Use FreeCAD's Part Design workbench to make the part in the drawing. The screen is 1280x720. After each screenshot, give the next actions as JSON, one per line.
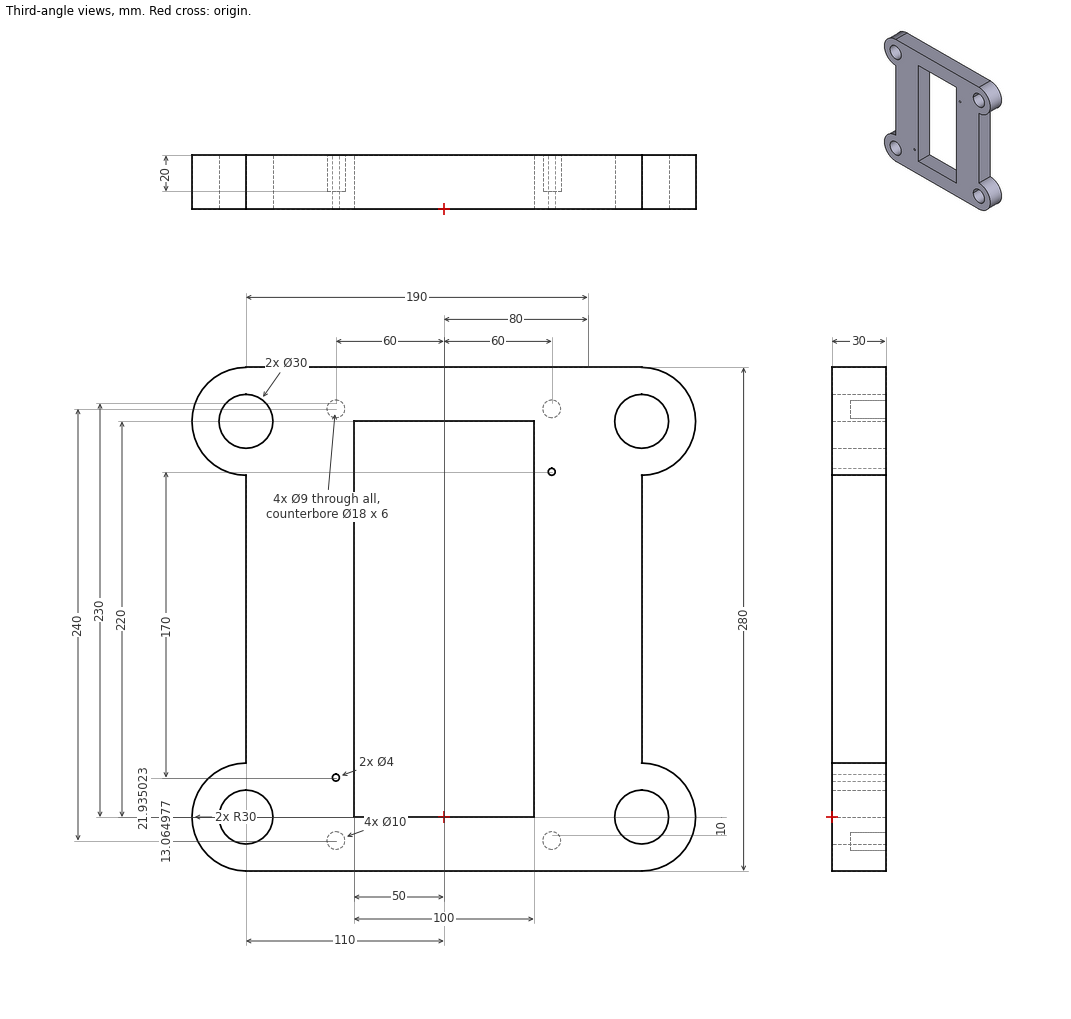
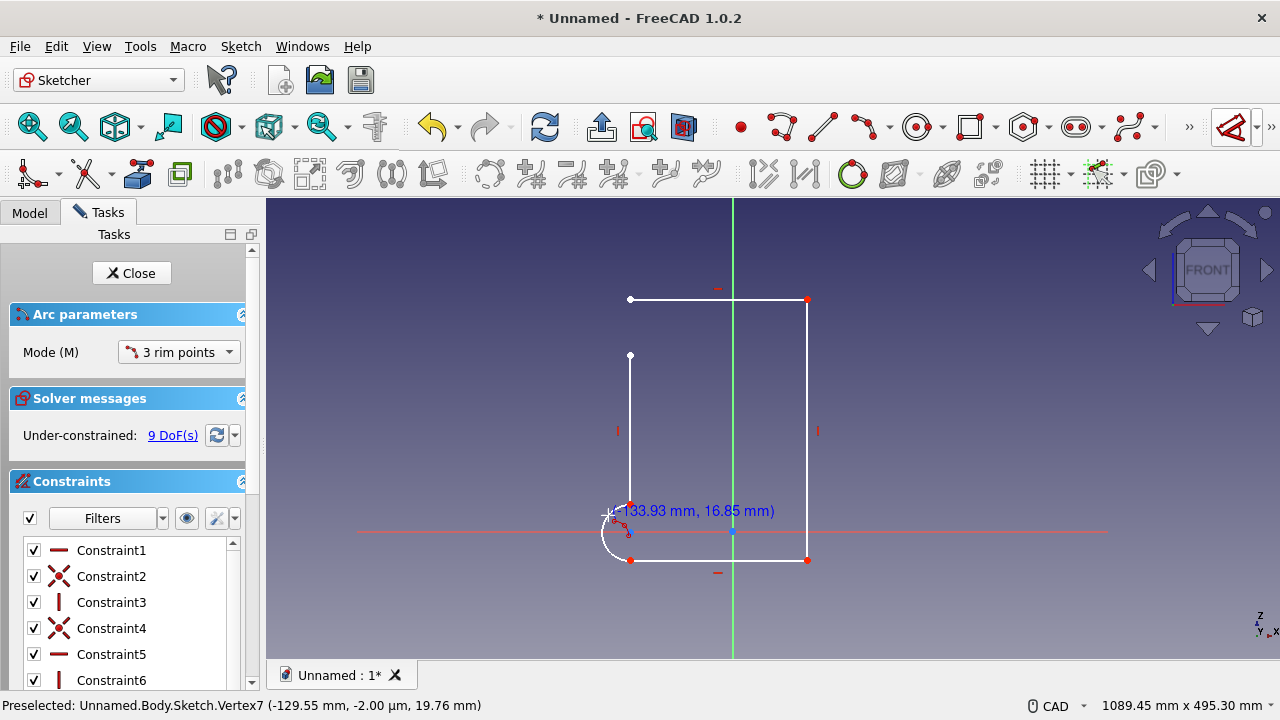
{"action": "left_click", "coordinate": [630, 356]}
{"action": "left_click", "coordinate": [630, 300]}
{"action": "left_click", "coordinate": [602, 327]}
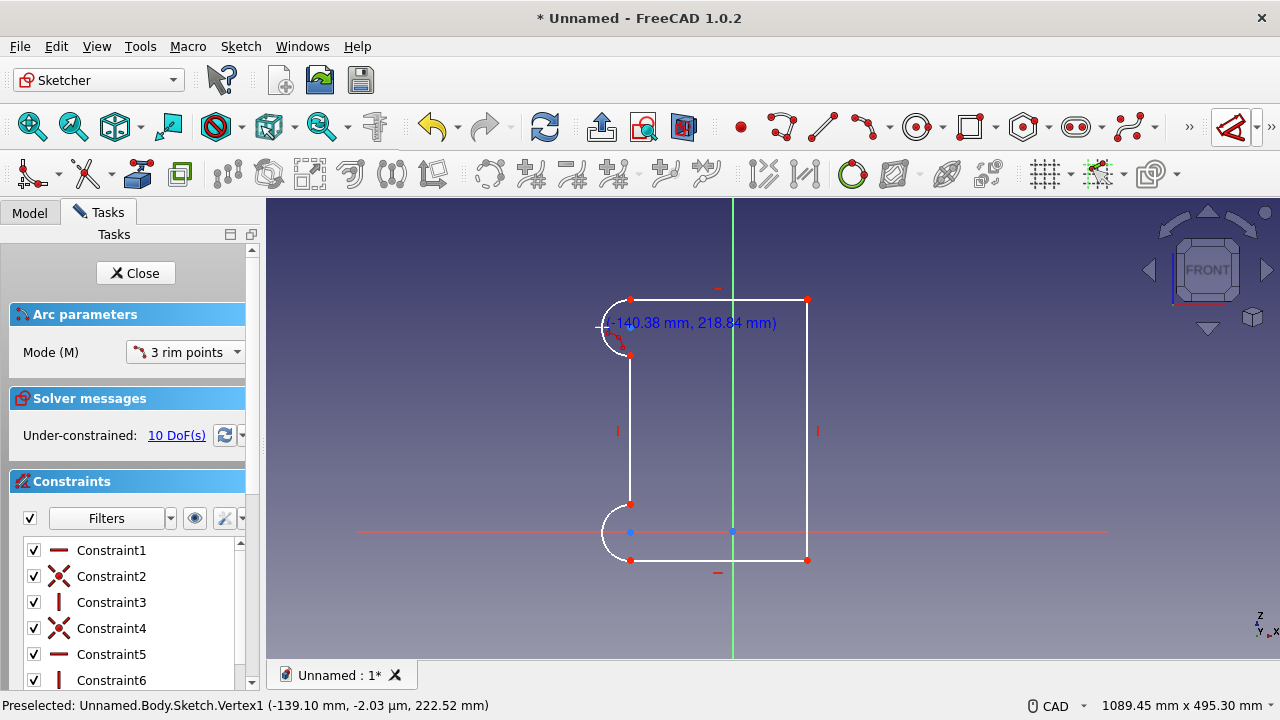
{"action": "left_click", "coordinate": [970, 128]}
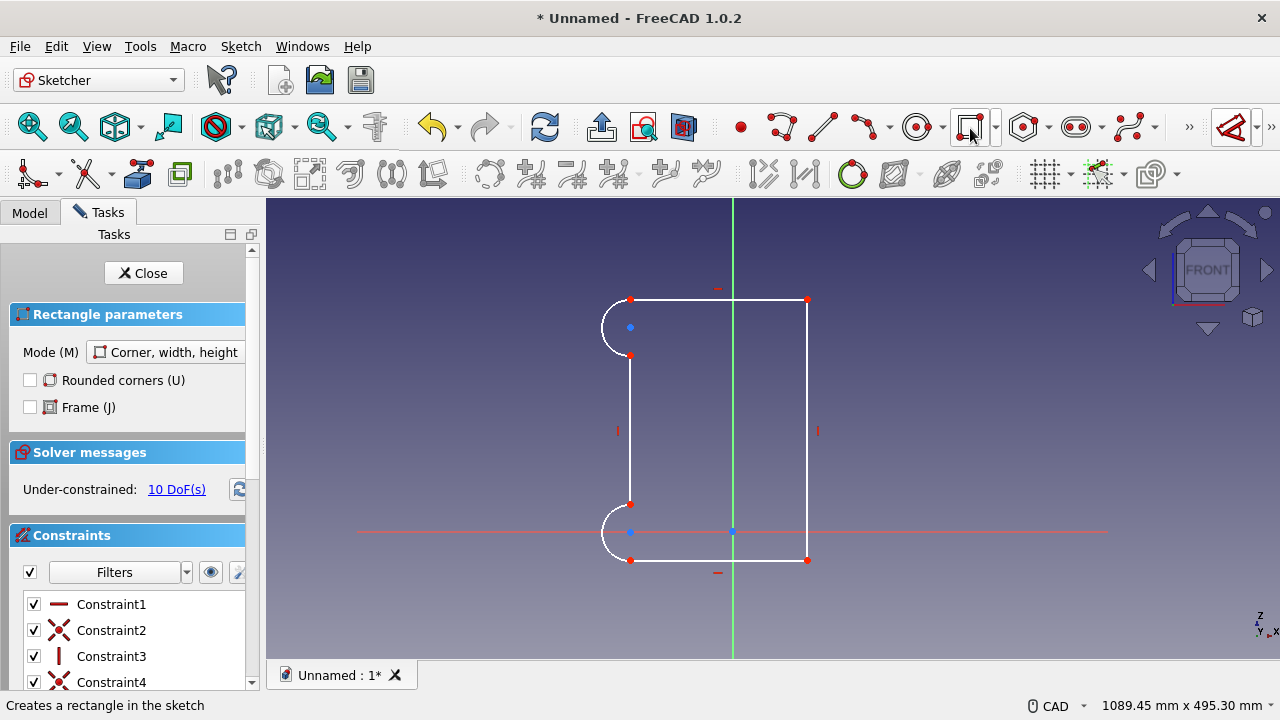
{"action": "left_click", "coordinate": [686, 327]}
{"action": "left_click", "coordinate": [779, 532]}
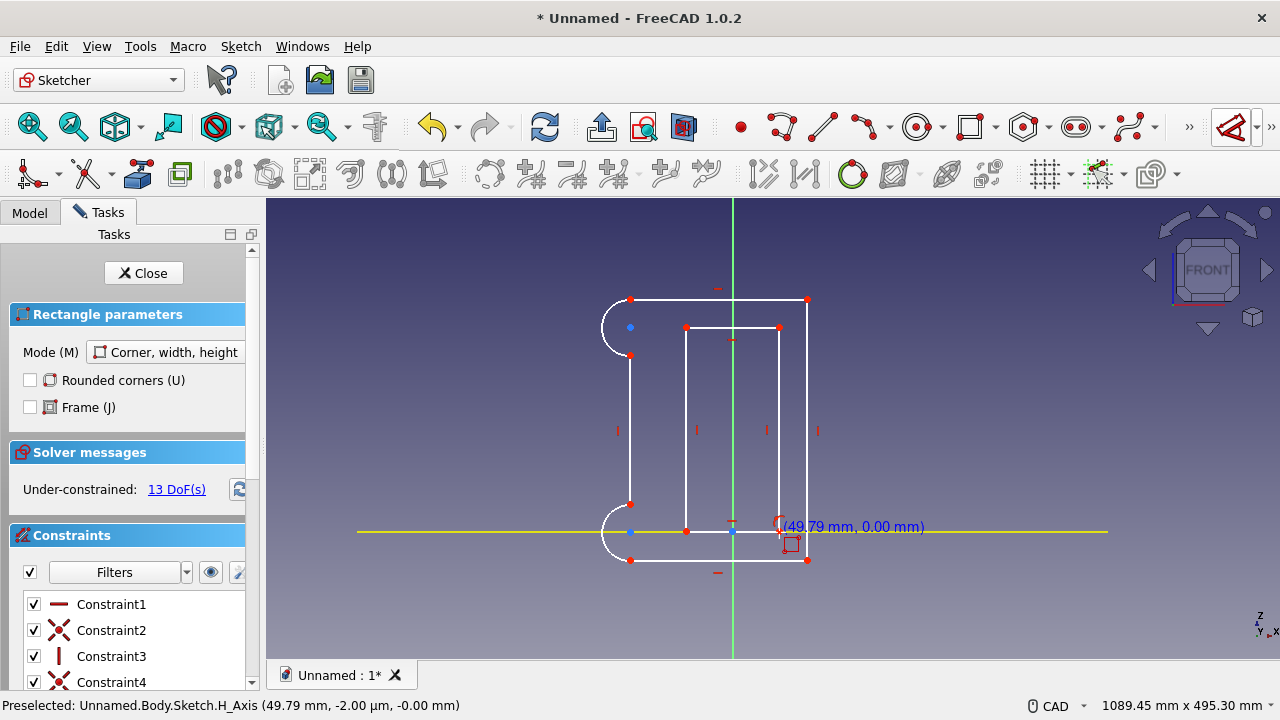
{"action": "left_click", "coordinate": [916, 128]}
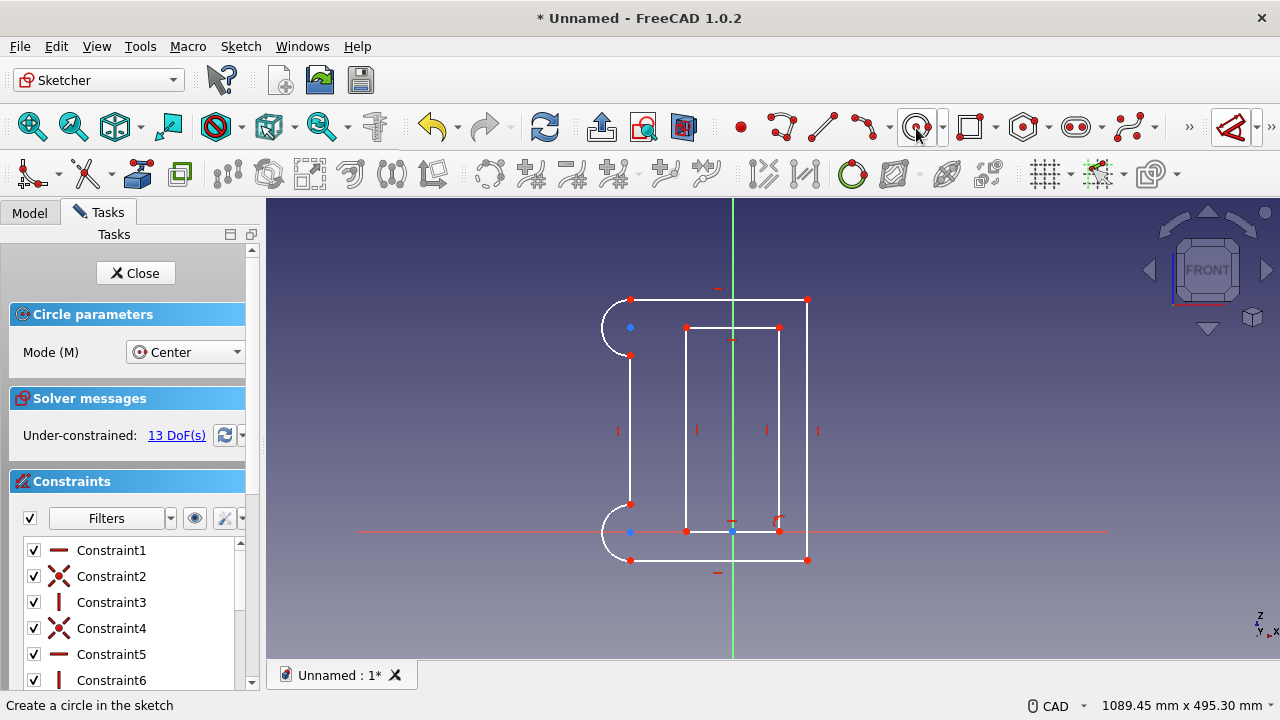
{"action": "scroll", "coordinate": [630, 327], "scroll_direction": "up", "scroll_amount": 3}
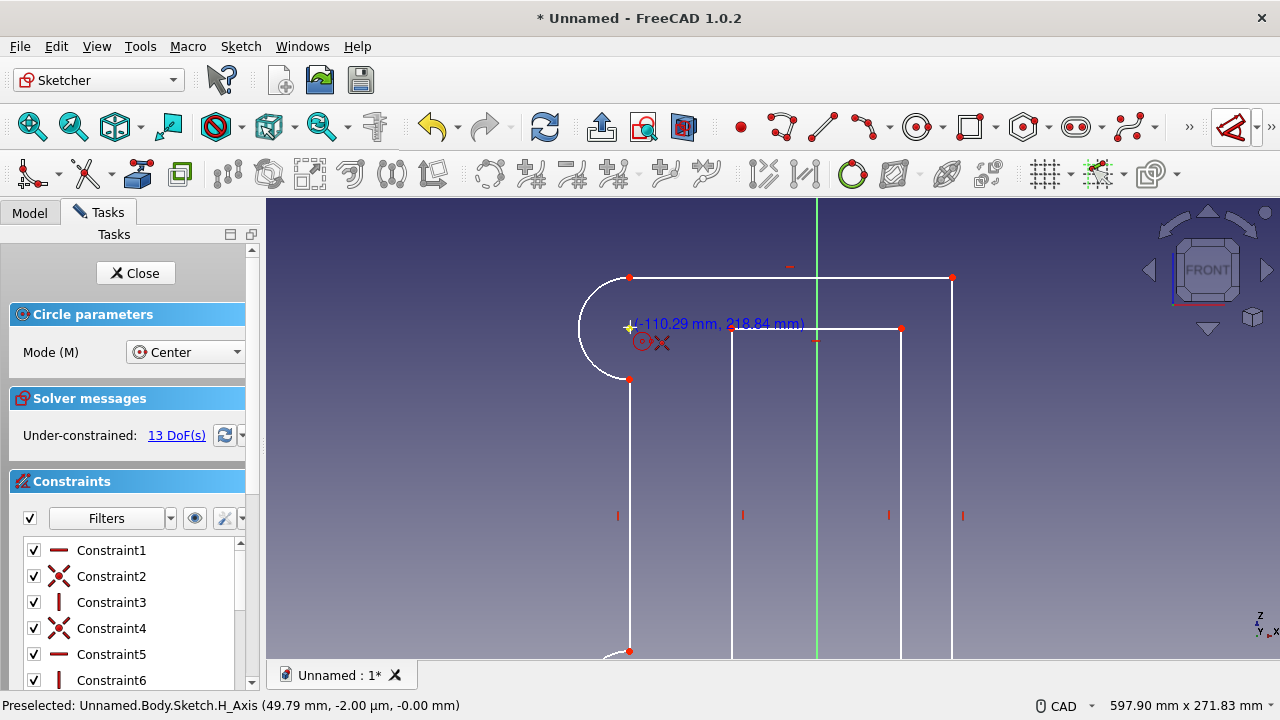
{"action": "left_click", "coordinate": [630, 327]}
{"action": "left_click", "coordinate": [648, 309]}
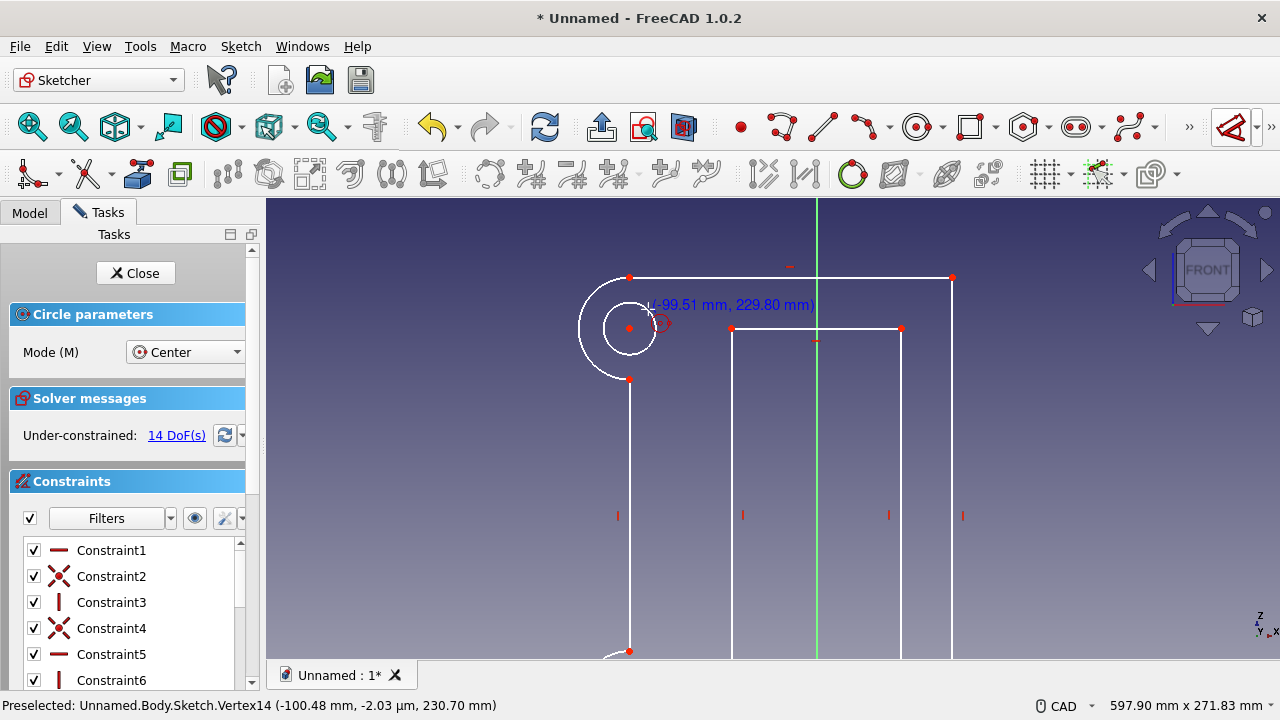
{"action": "scroll", "coordinate": [630, 326], "scroll_direction": "down", "scroll_amount": 3}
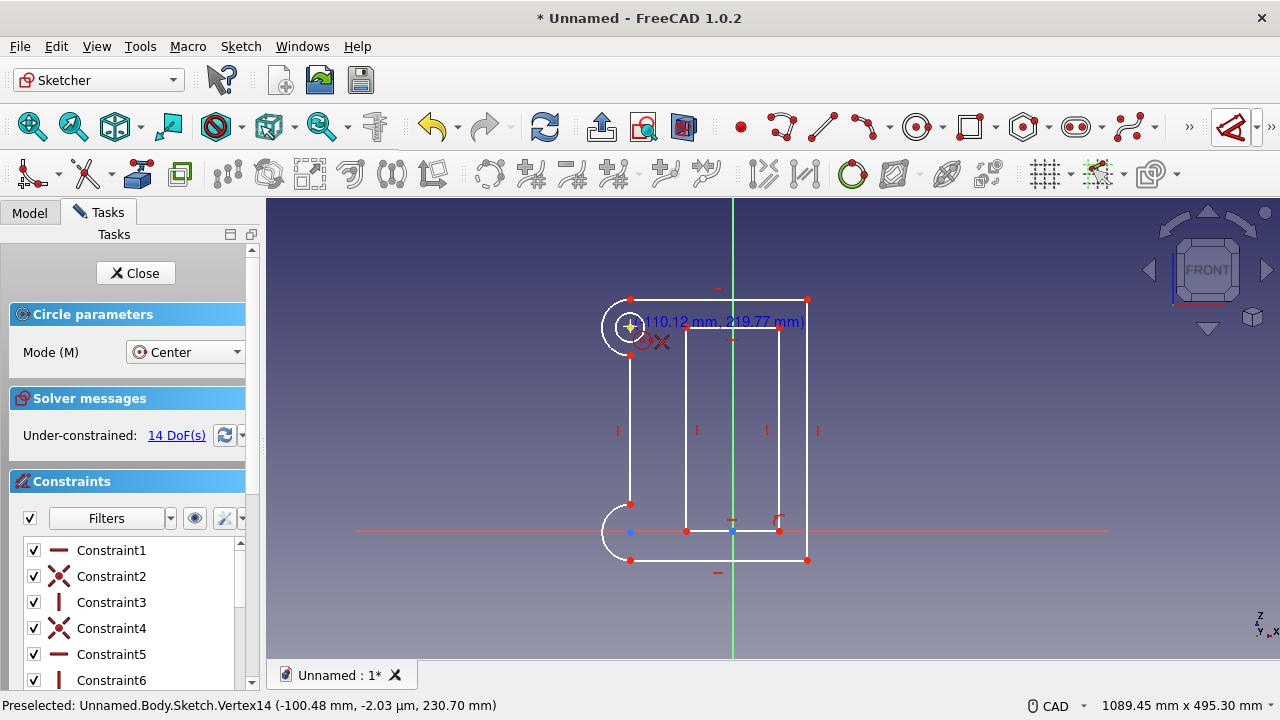
{"action": "scroll", "coordinate": [630, 531], "scroll_direction": "up", "scroll_amount": 3}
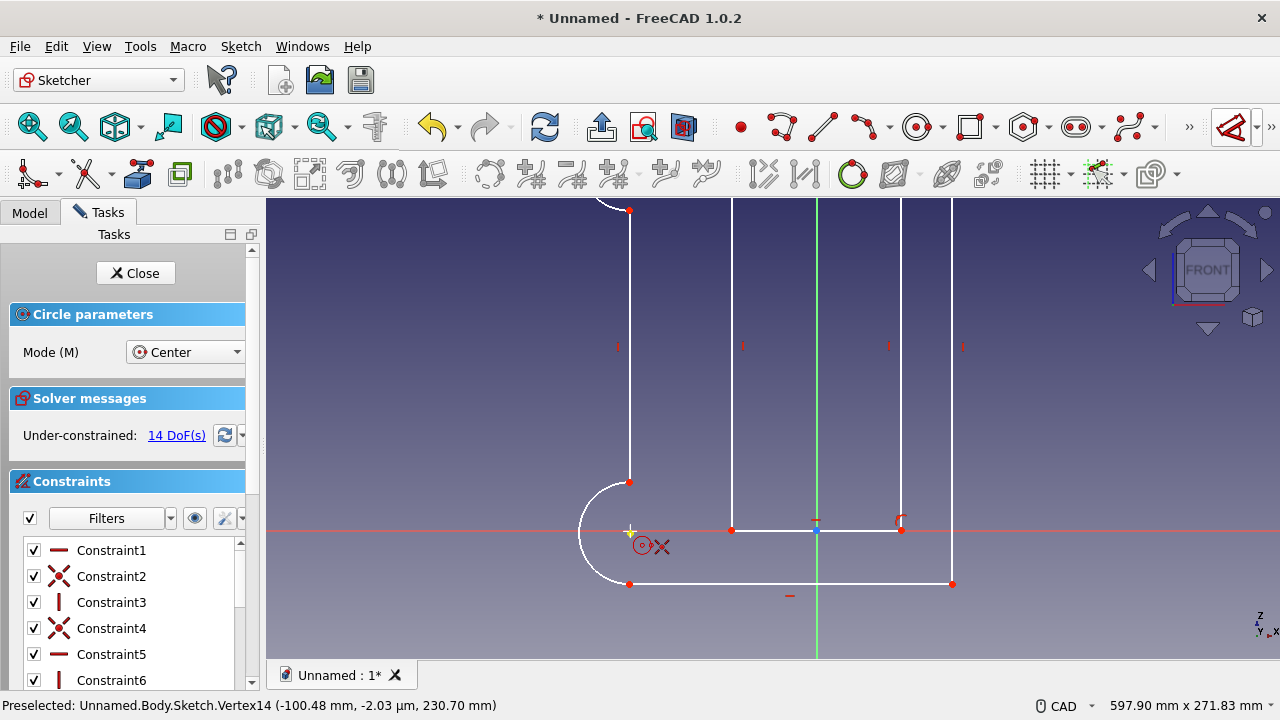
{"action": "left_click", "coordinate": [630, 531]}
{"action": "left_click", "coordinate": [648, 513]}
{"action": "key", "text": "Escape"}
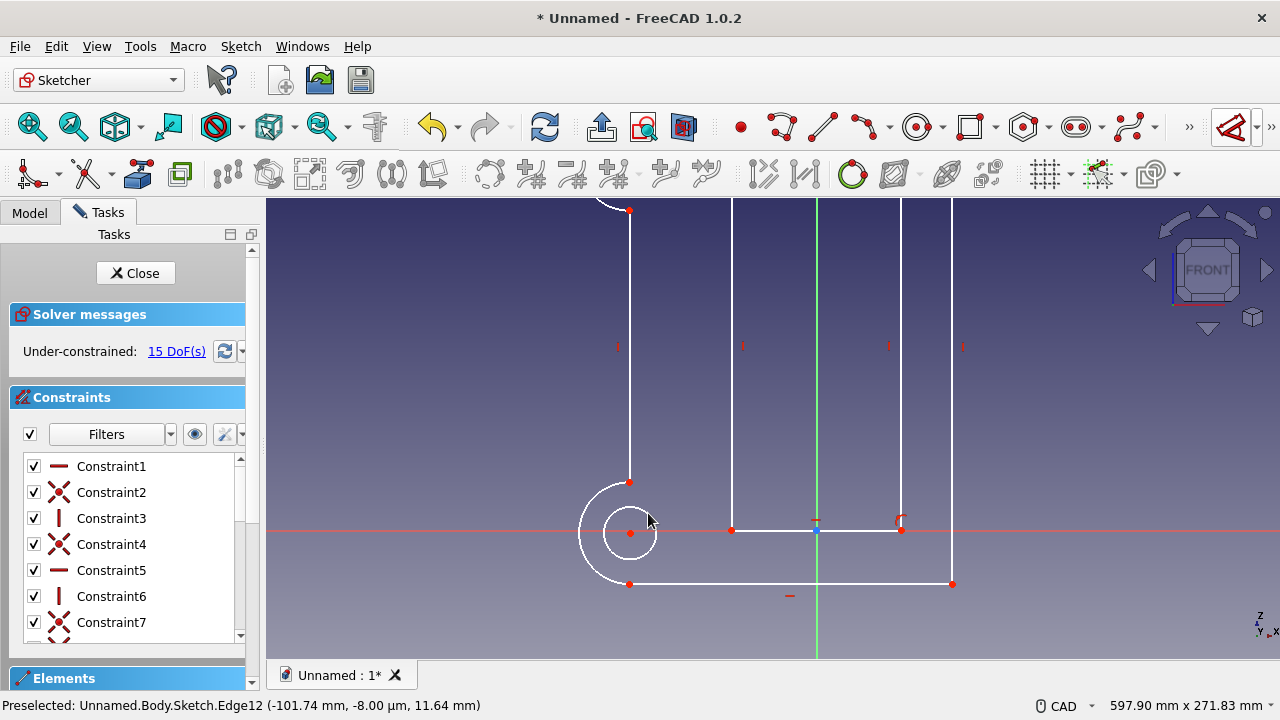
{"action": "scroll", "coordinate": [630, 531], "scroll_direction": "down", "scroll_amount": 3}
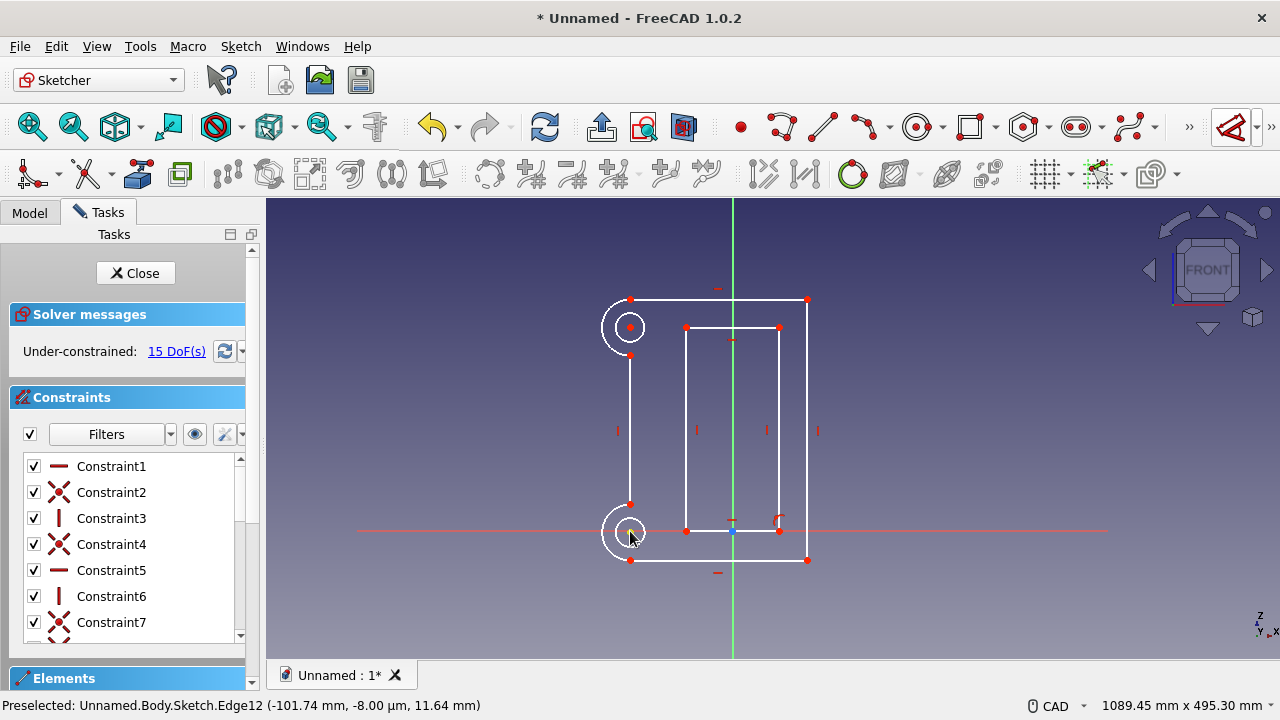
{"action": "left_click", "coordinate": [683, 300]}